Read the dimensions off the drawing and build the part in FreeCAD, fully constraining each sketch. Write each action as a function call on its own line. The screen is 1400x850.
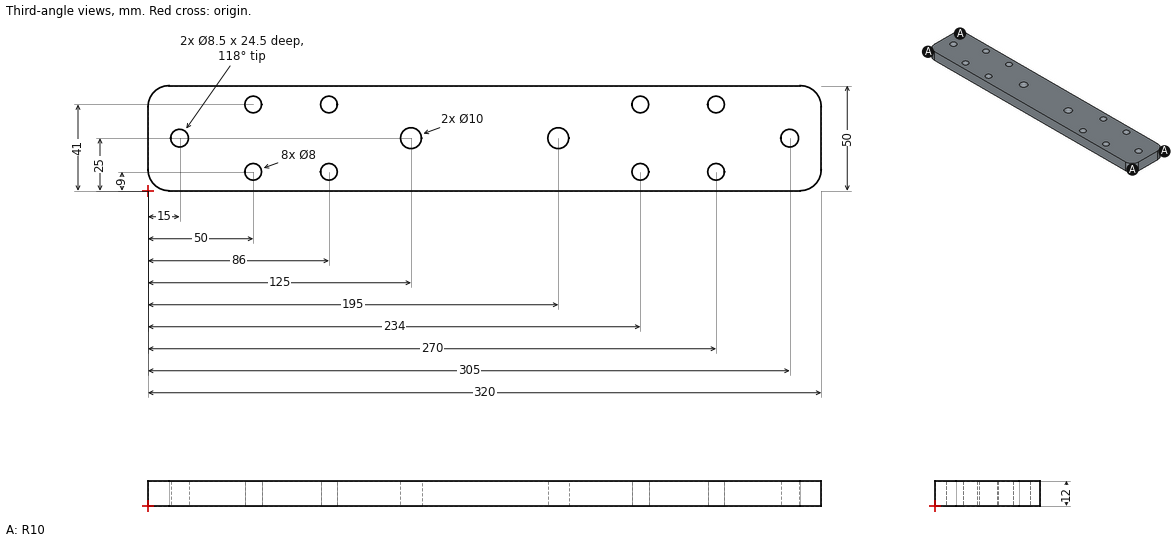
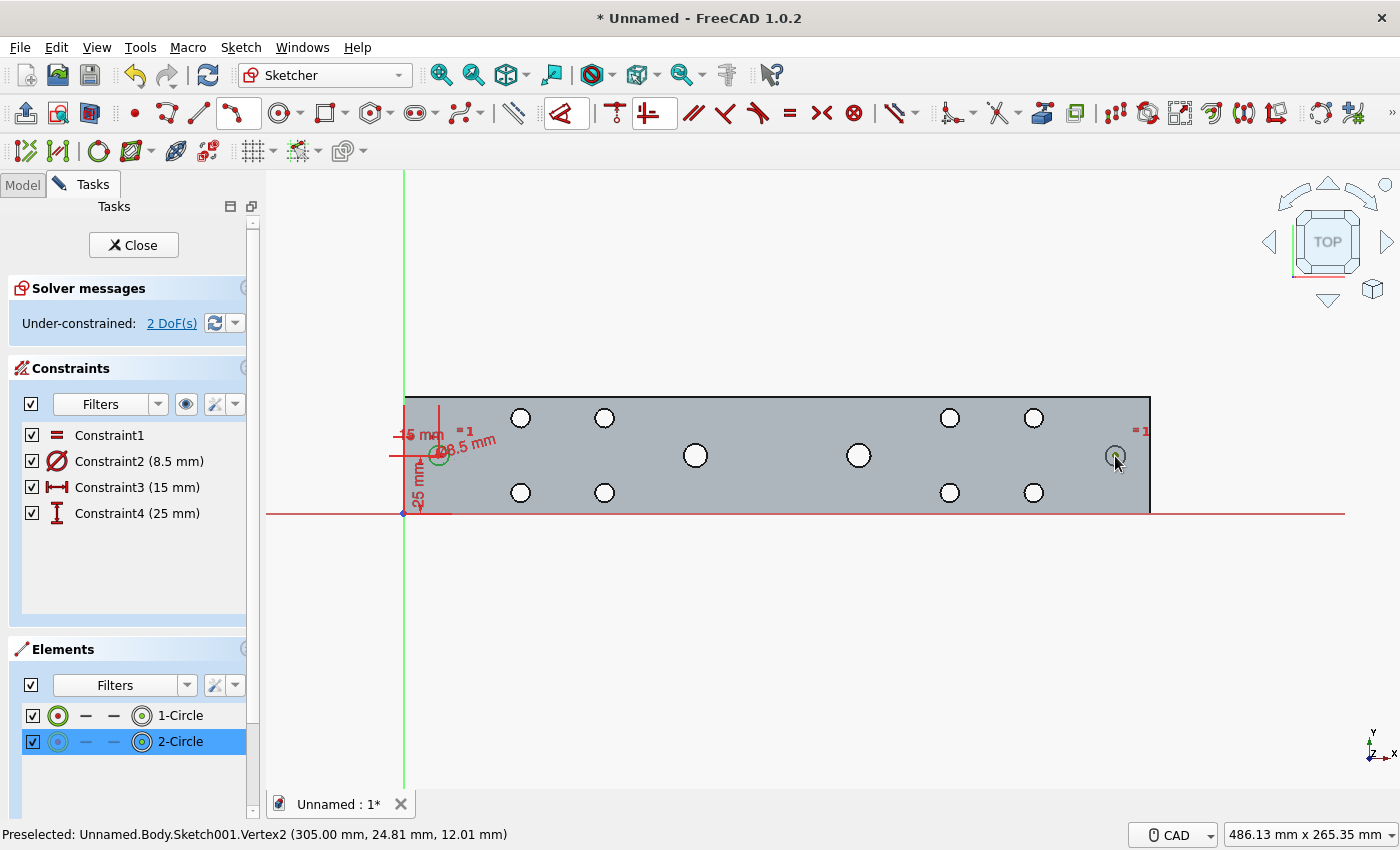
key(i)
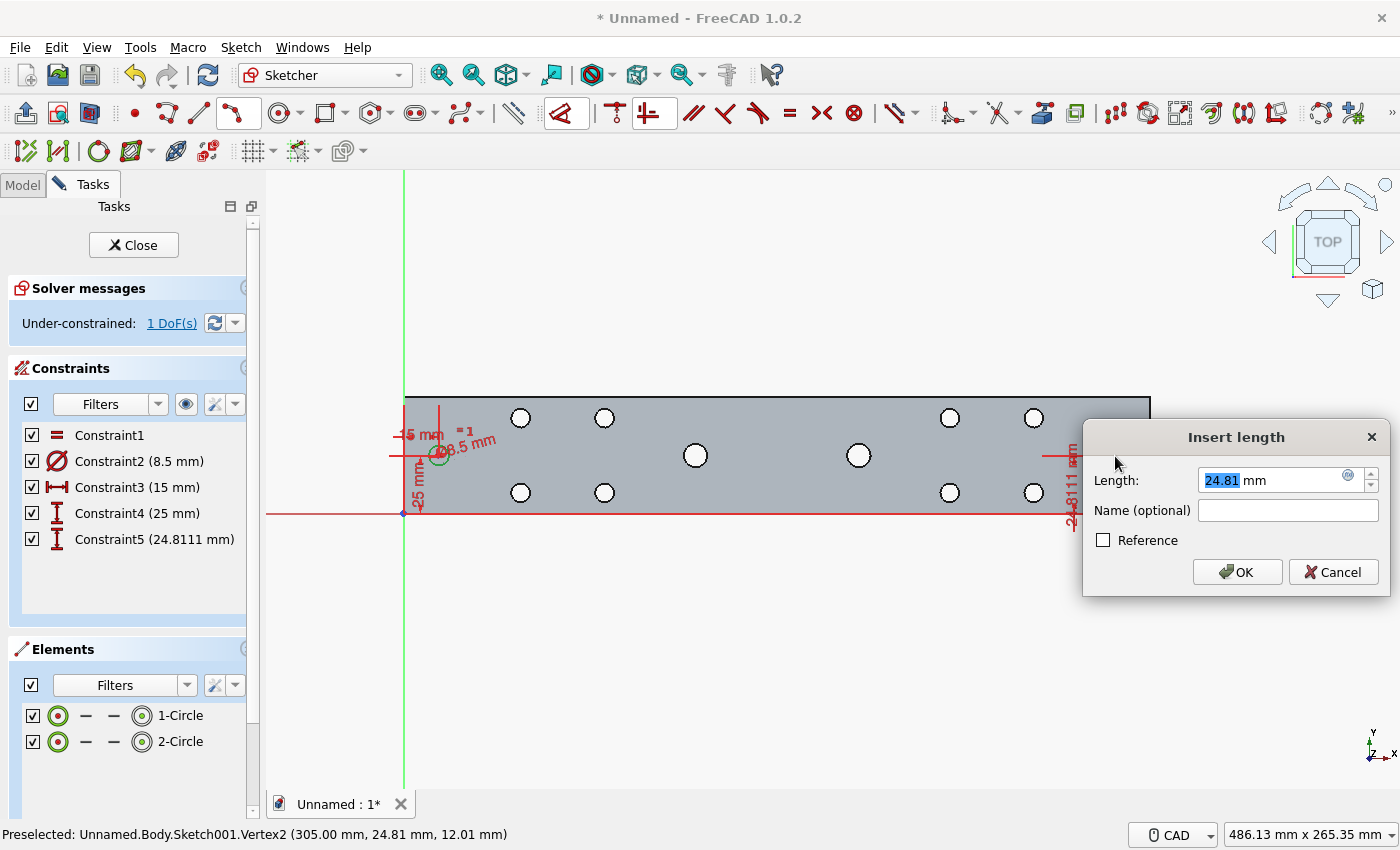
text(25)
key(Return)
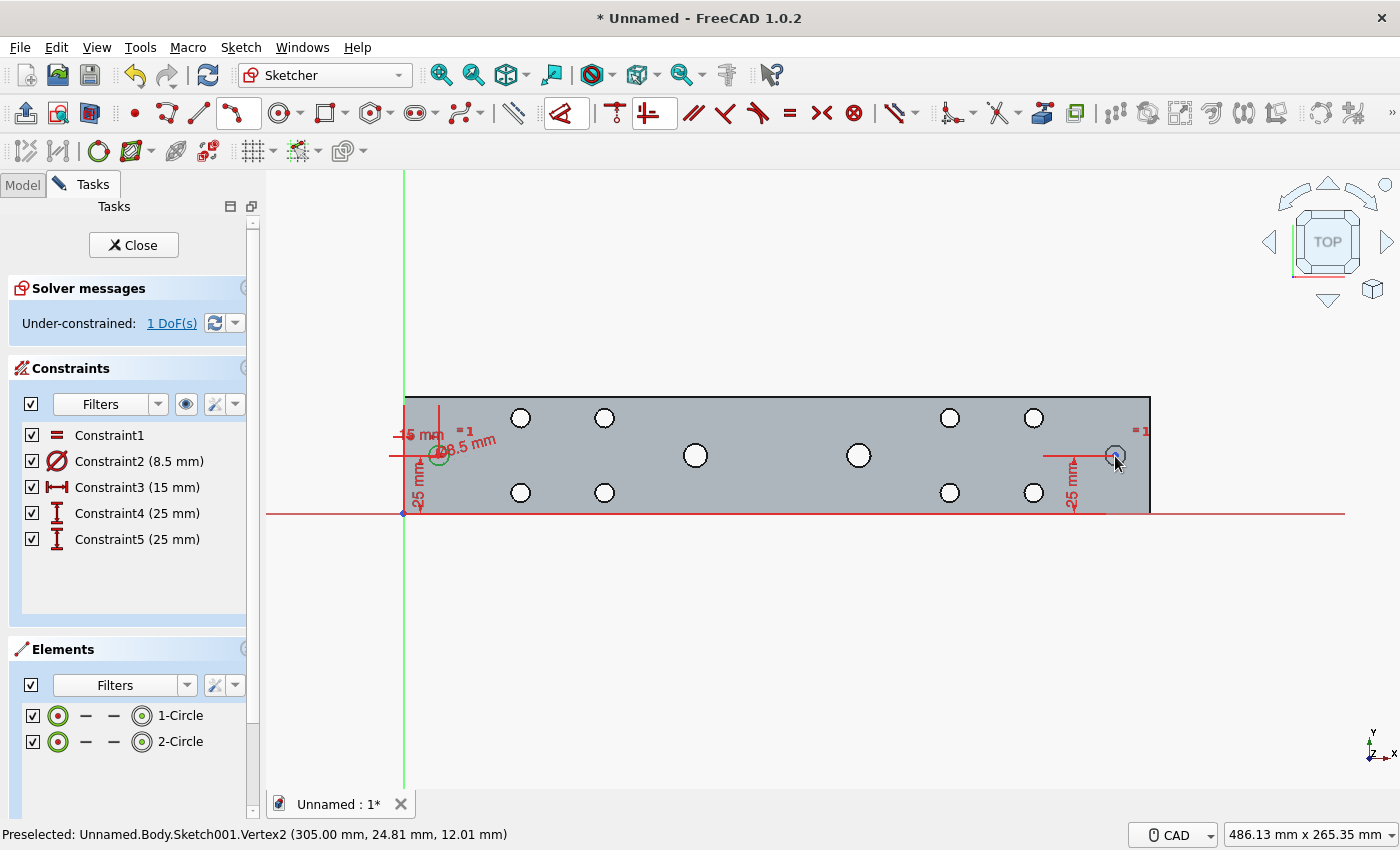
click(1115, 456)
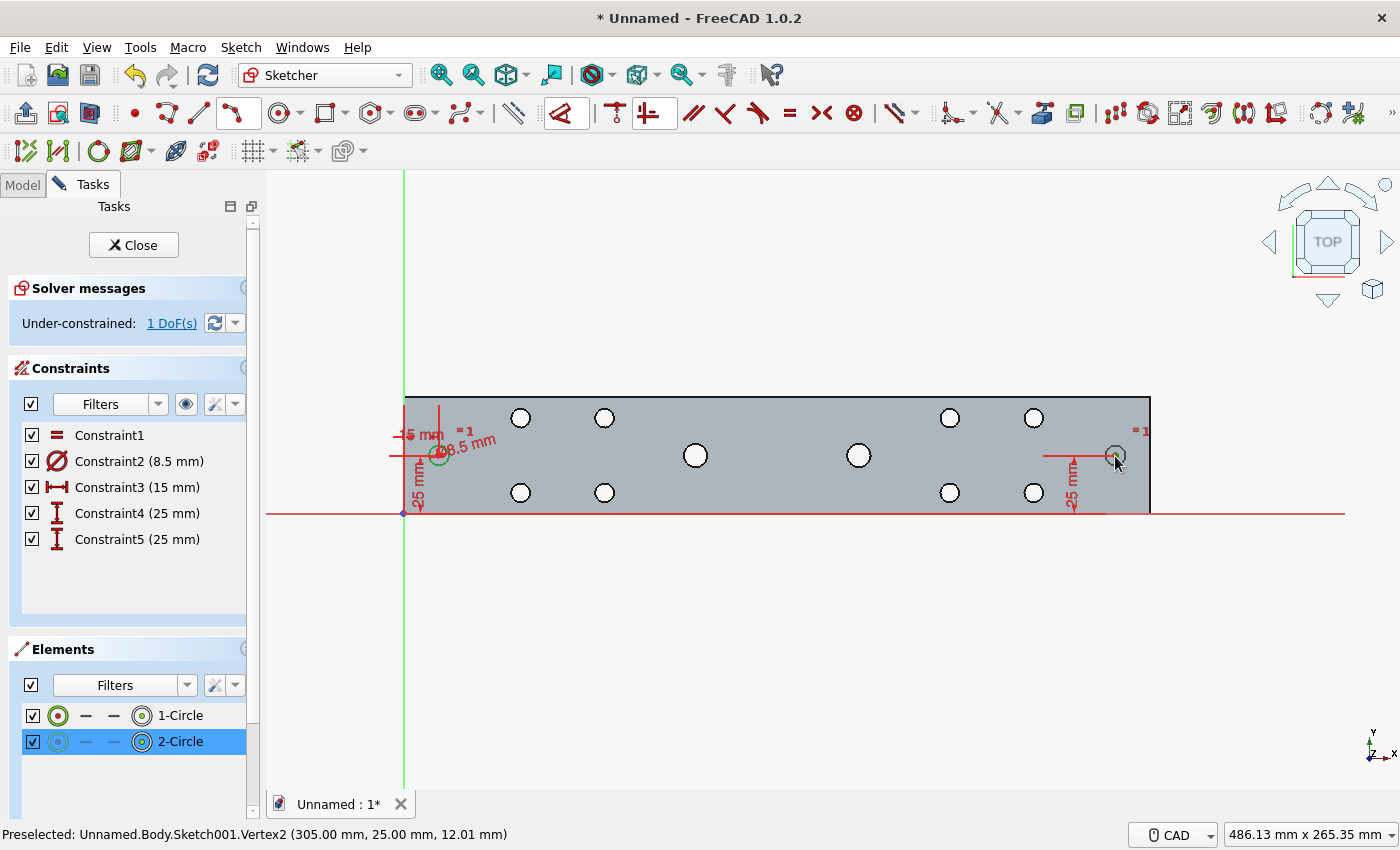
key(l)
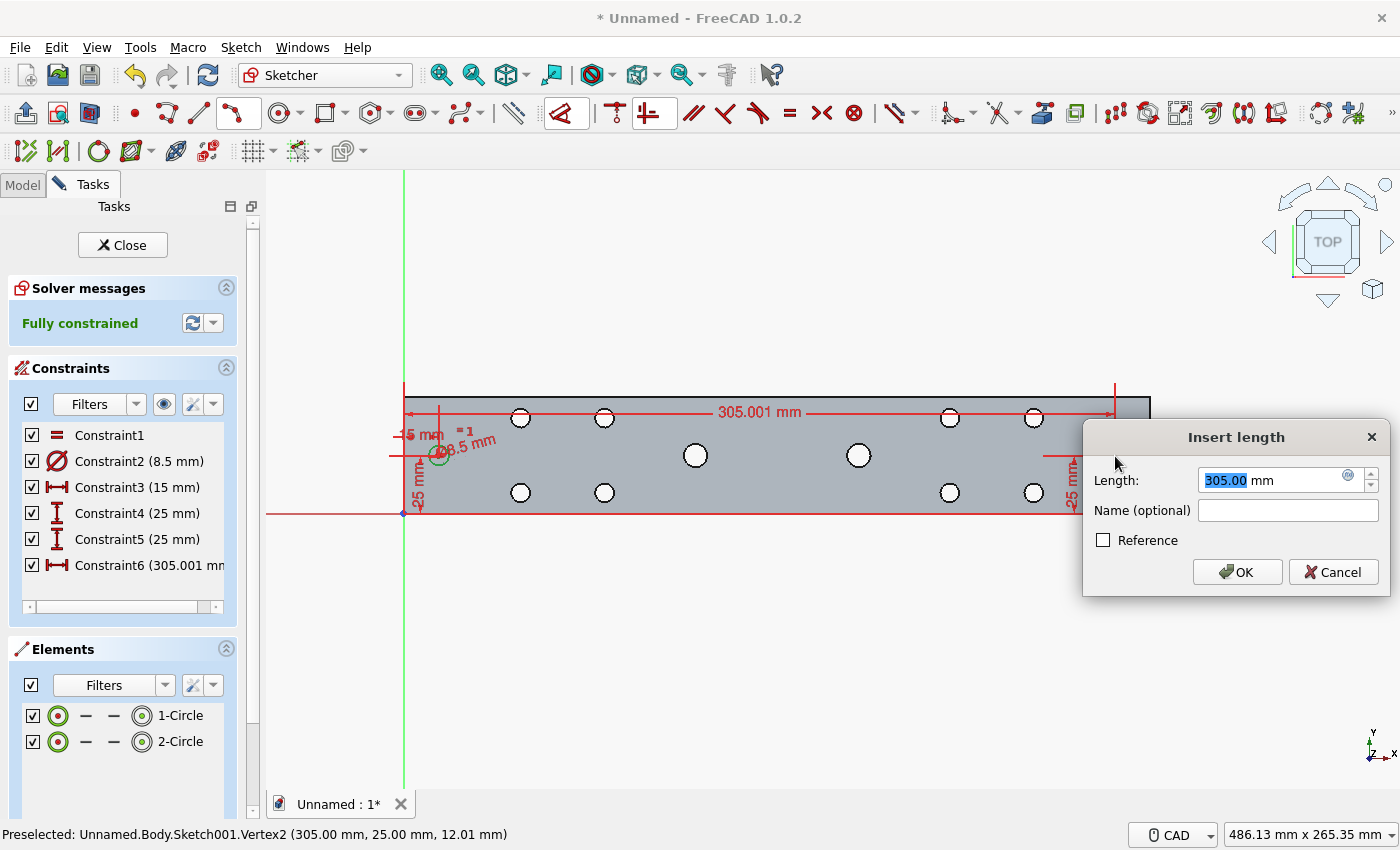
text(305)
key(Return)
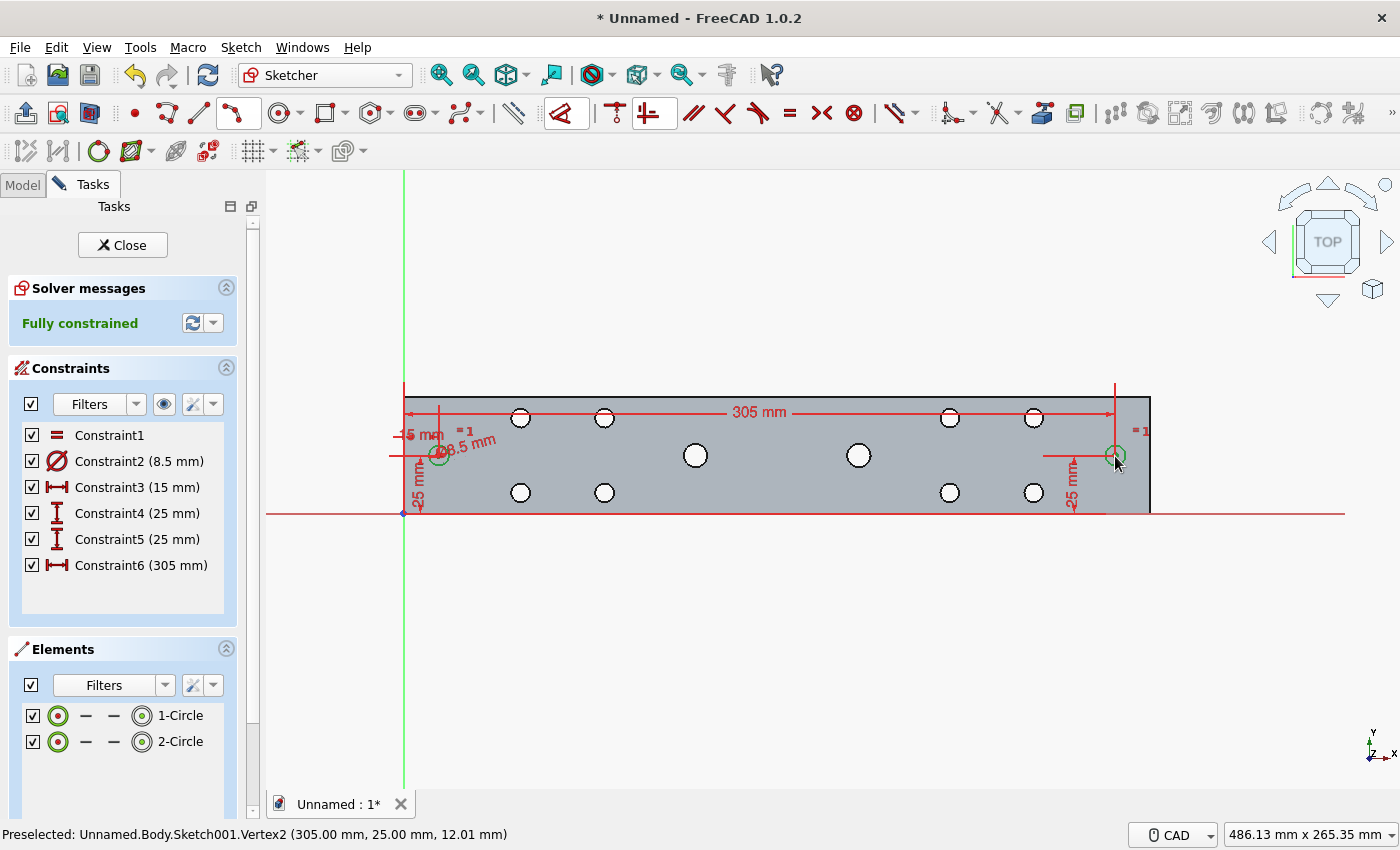
click(123, 245)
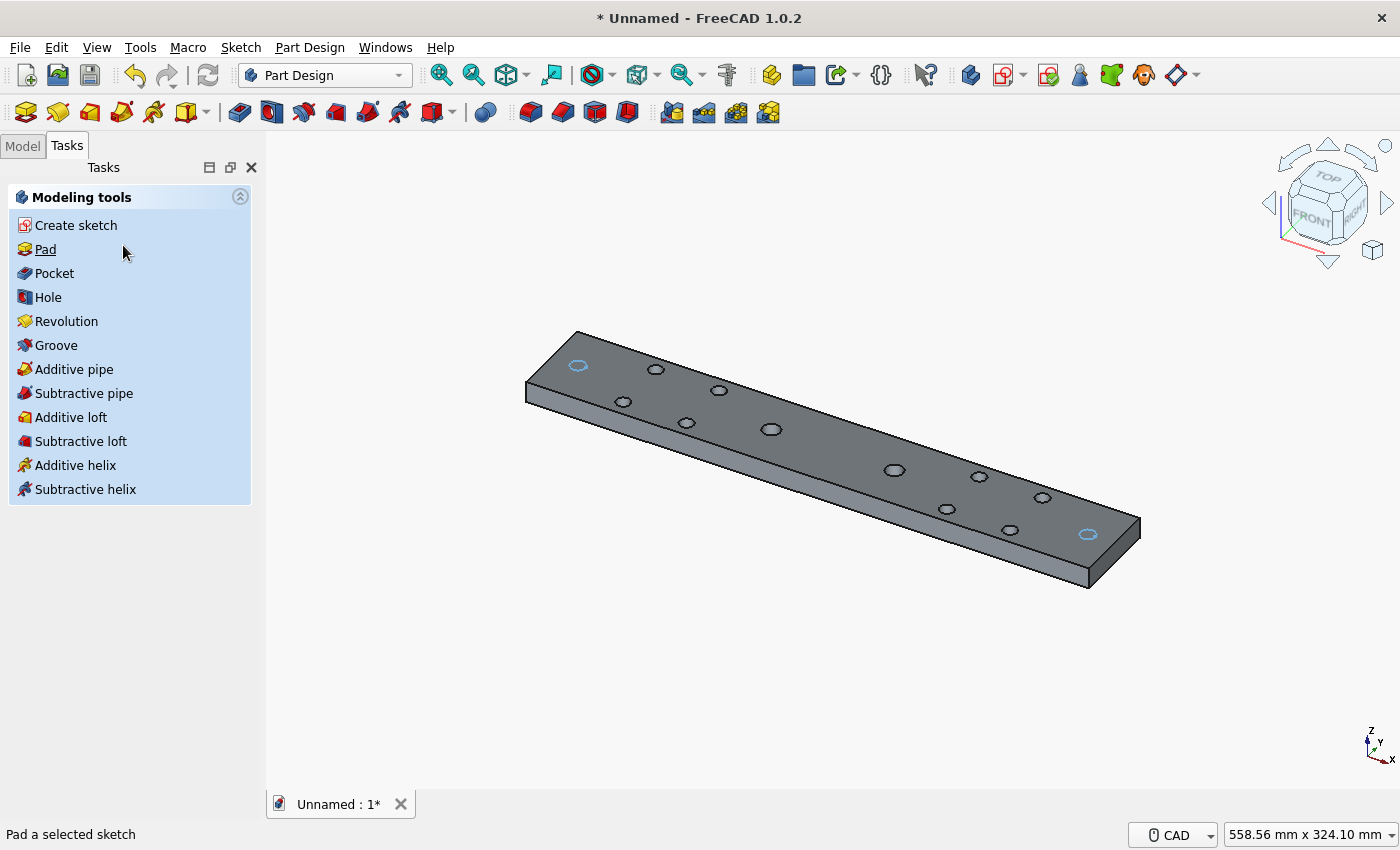
click(272, 112)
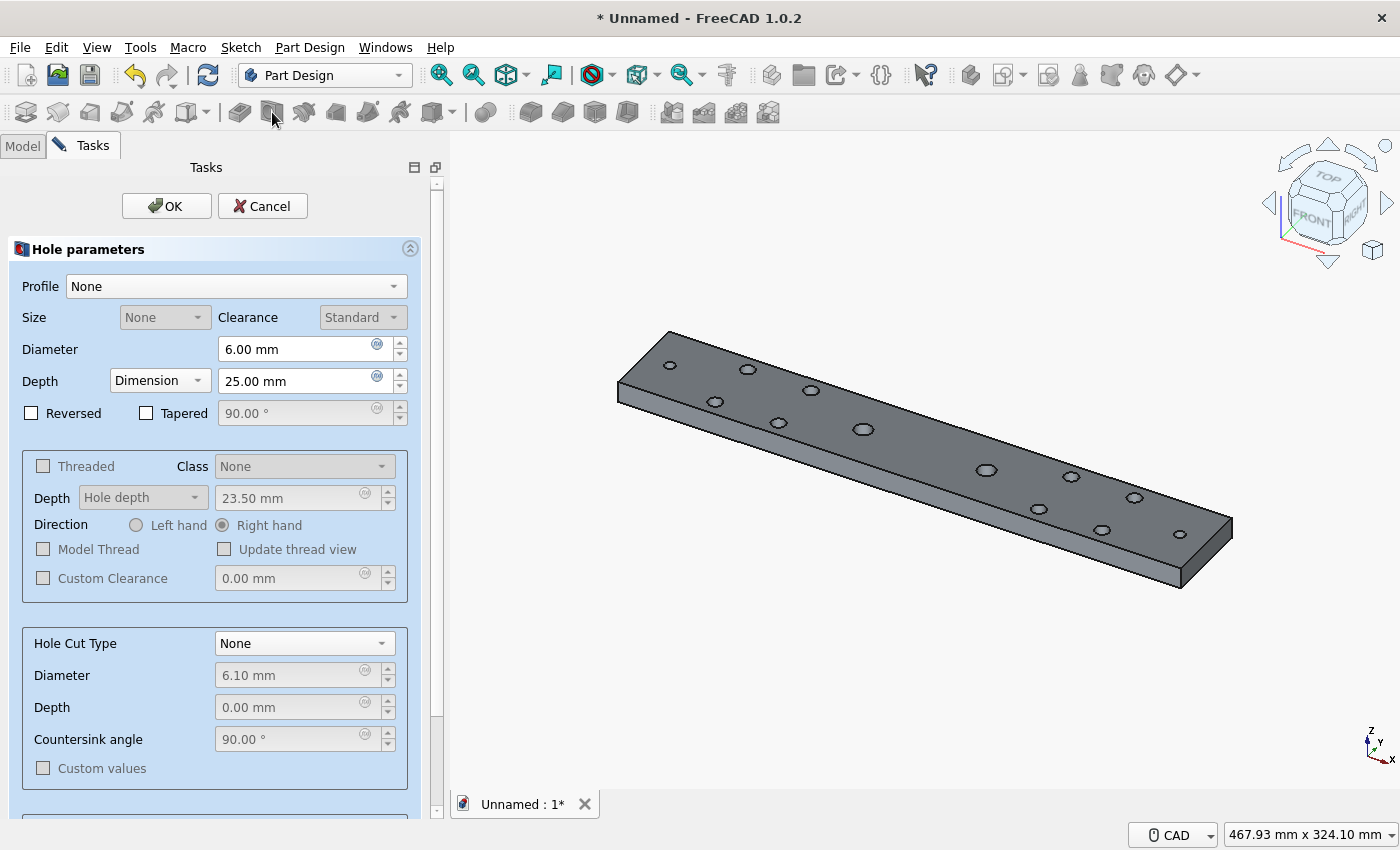
triple_click(305, 349)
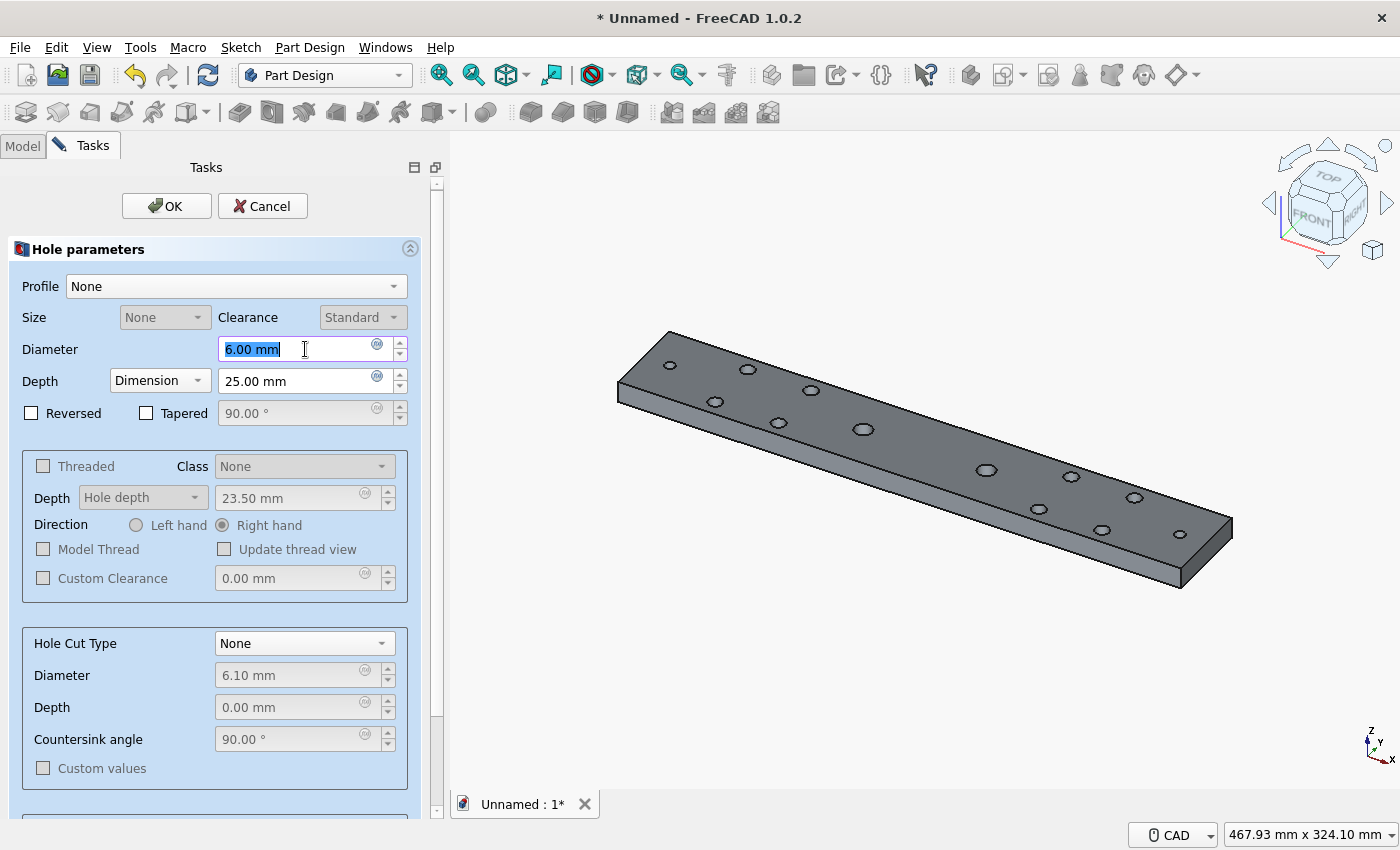
text(8.5)
key(Tab)